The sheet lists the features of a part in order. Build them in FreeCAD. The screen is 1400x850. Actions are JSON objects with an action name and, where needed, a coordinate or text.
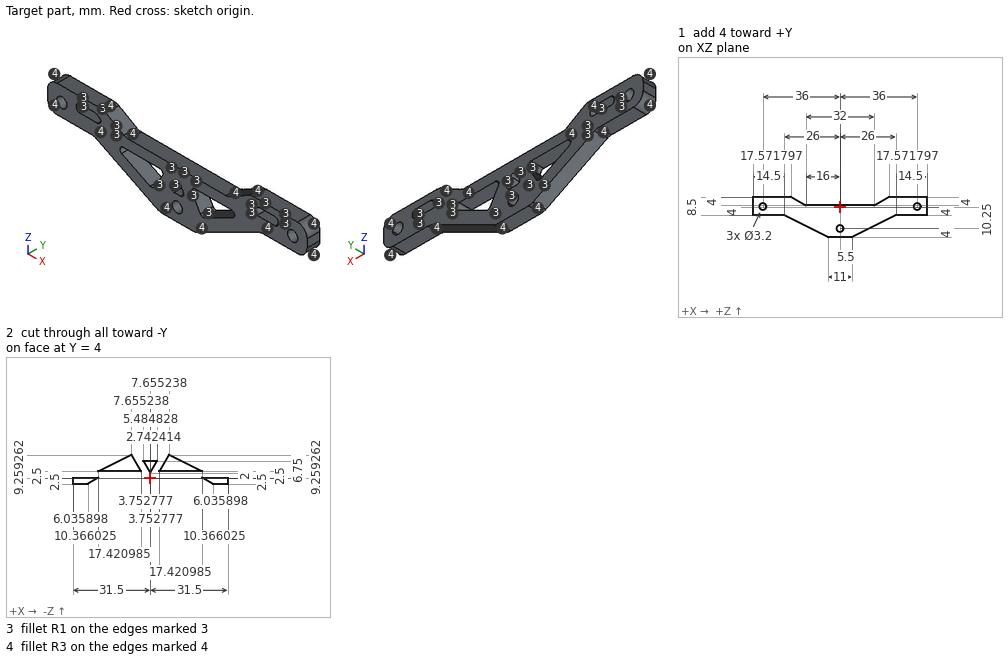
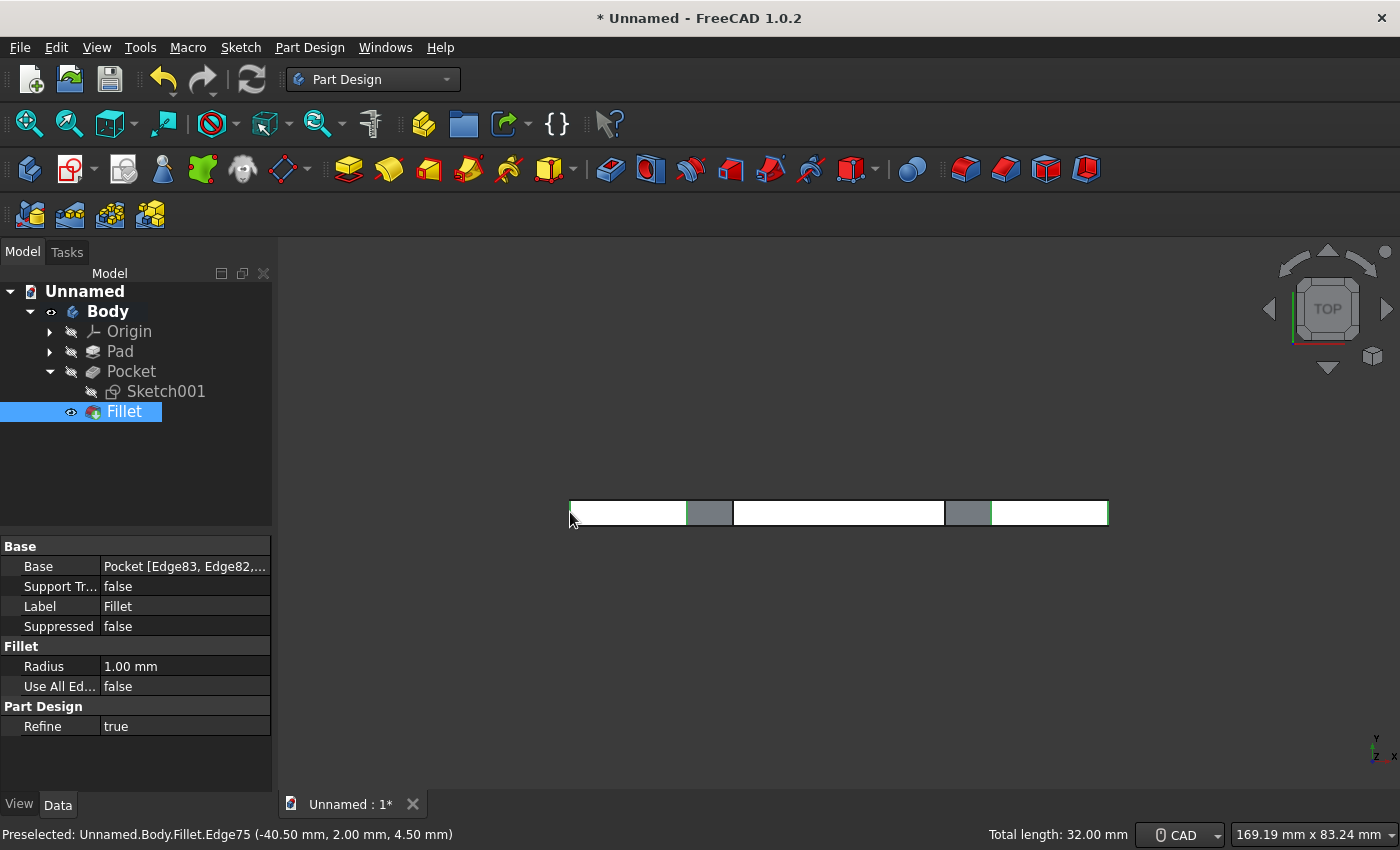
{"action": "key", "text": "1"}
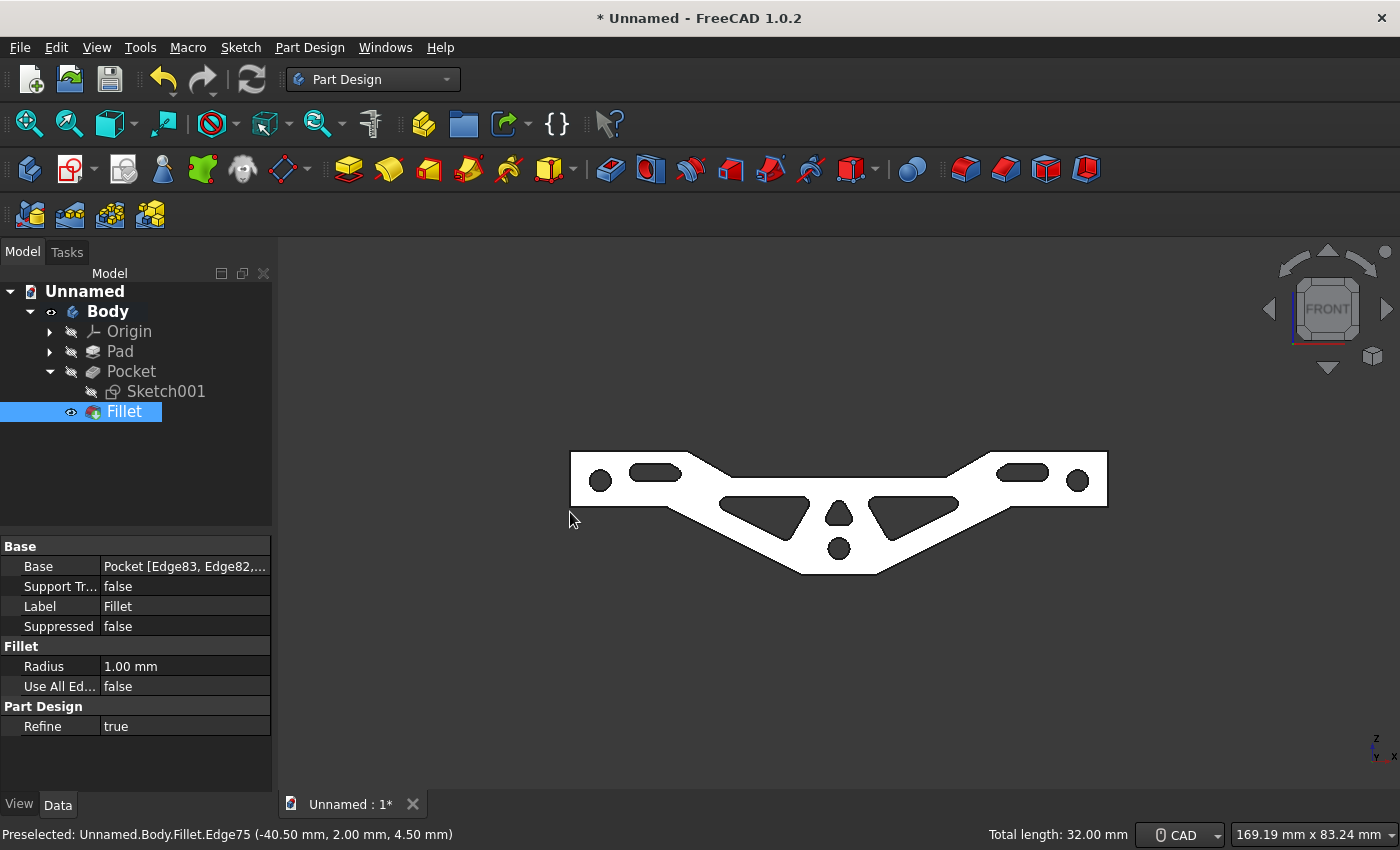
{"action": "key", "text": "3"}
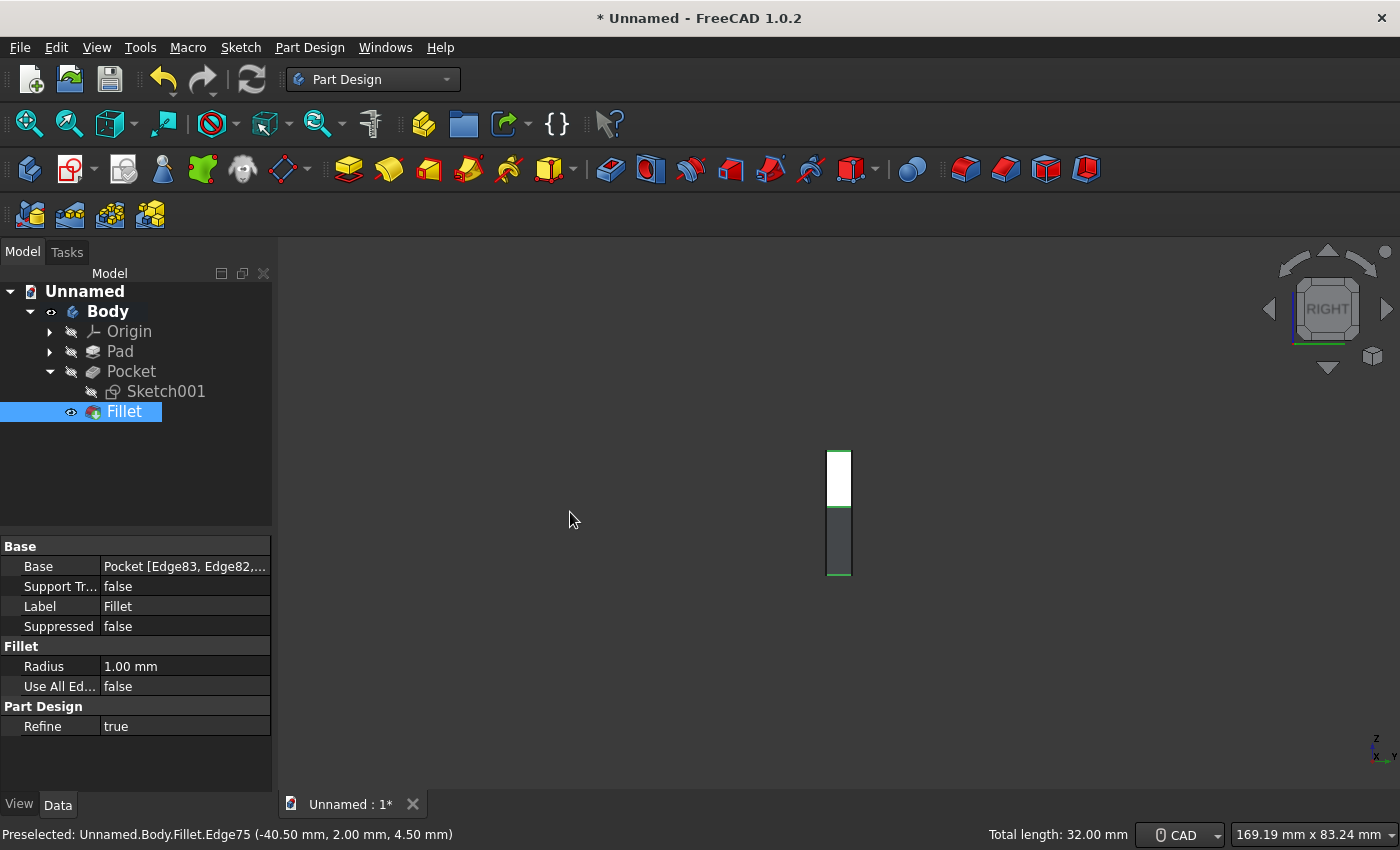
{"action": "left_click", "coordinate": [30, 124]}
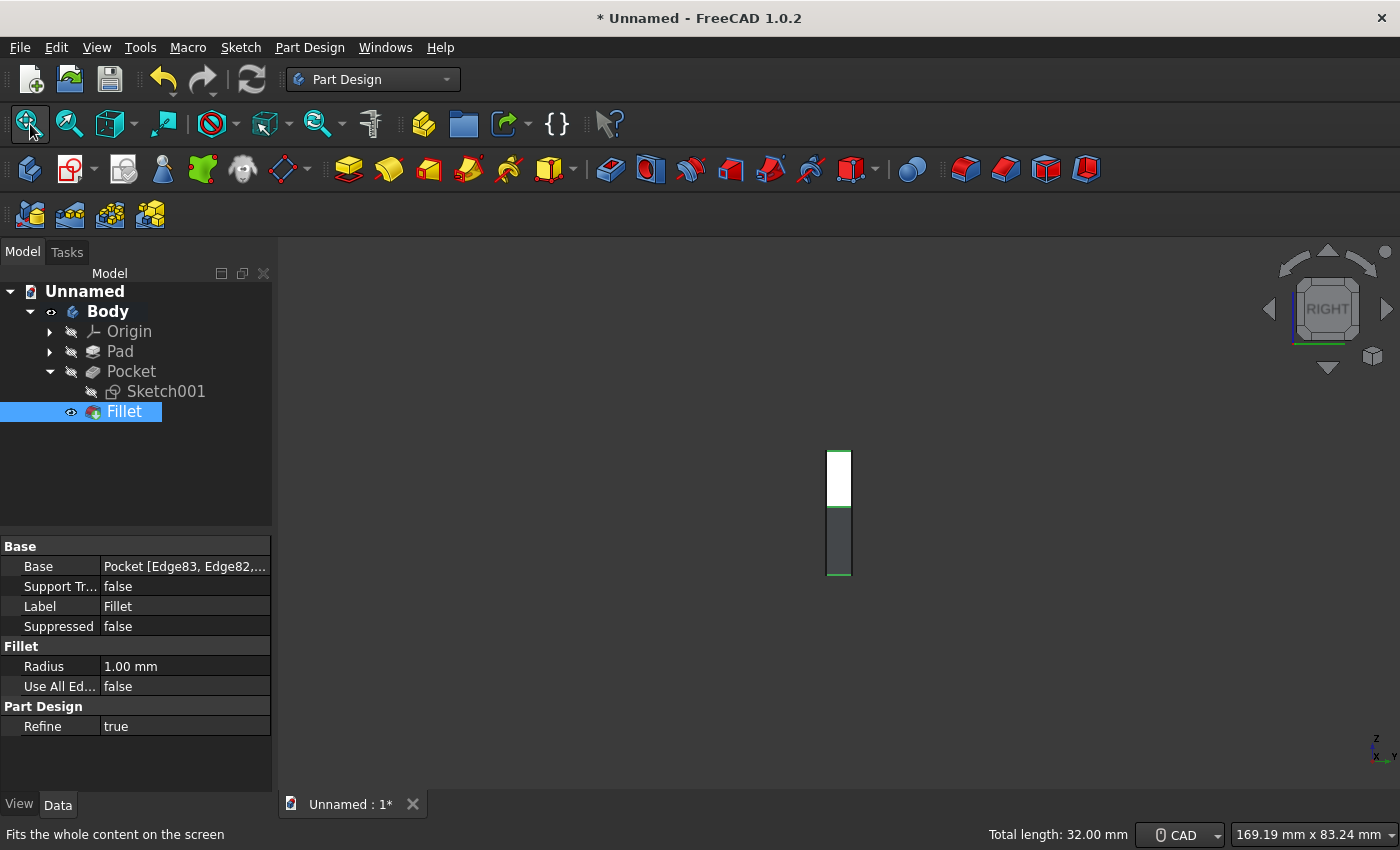
{"action": "key", "text": "5"}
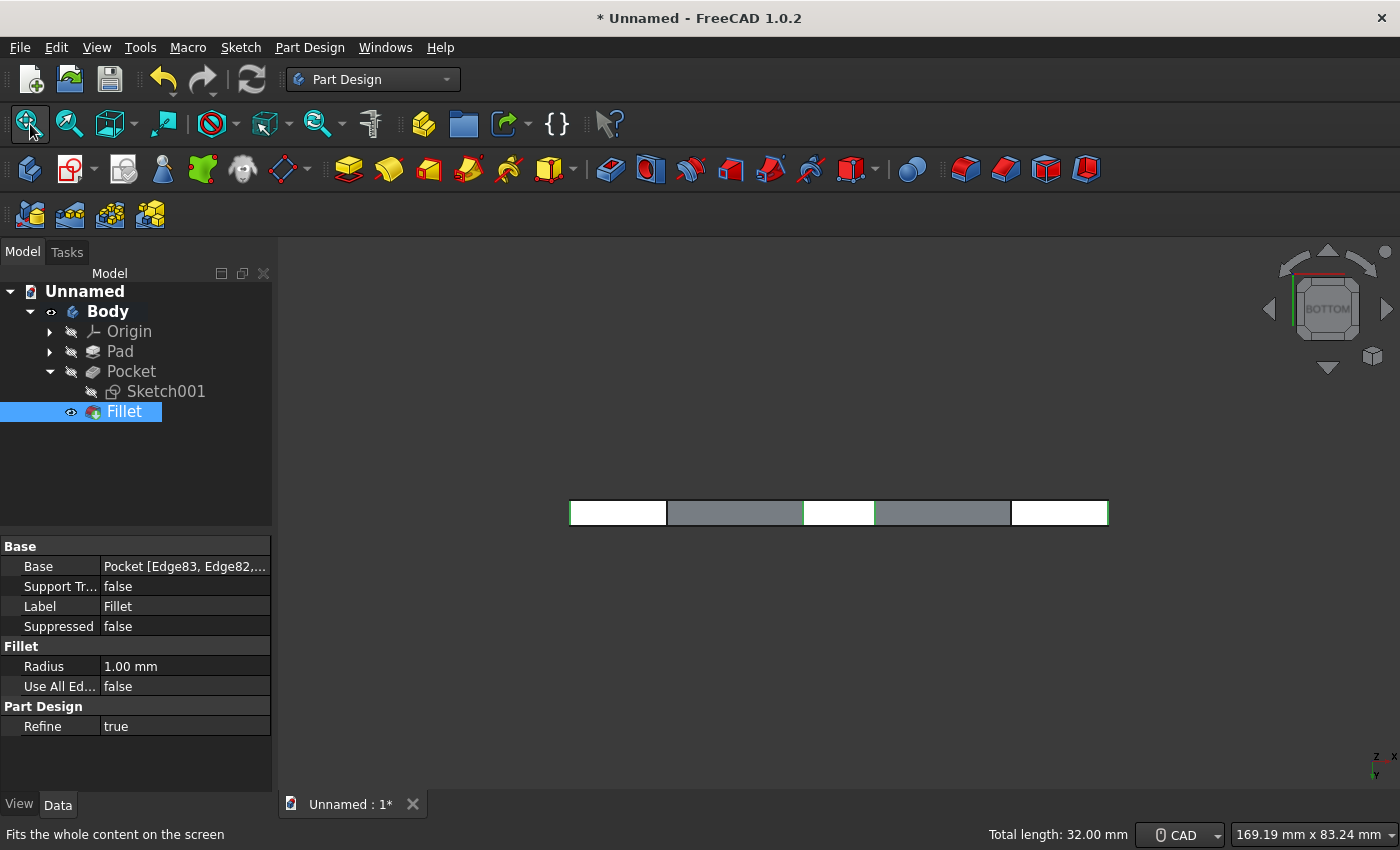
{"action": "key", "text": "4"}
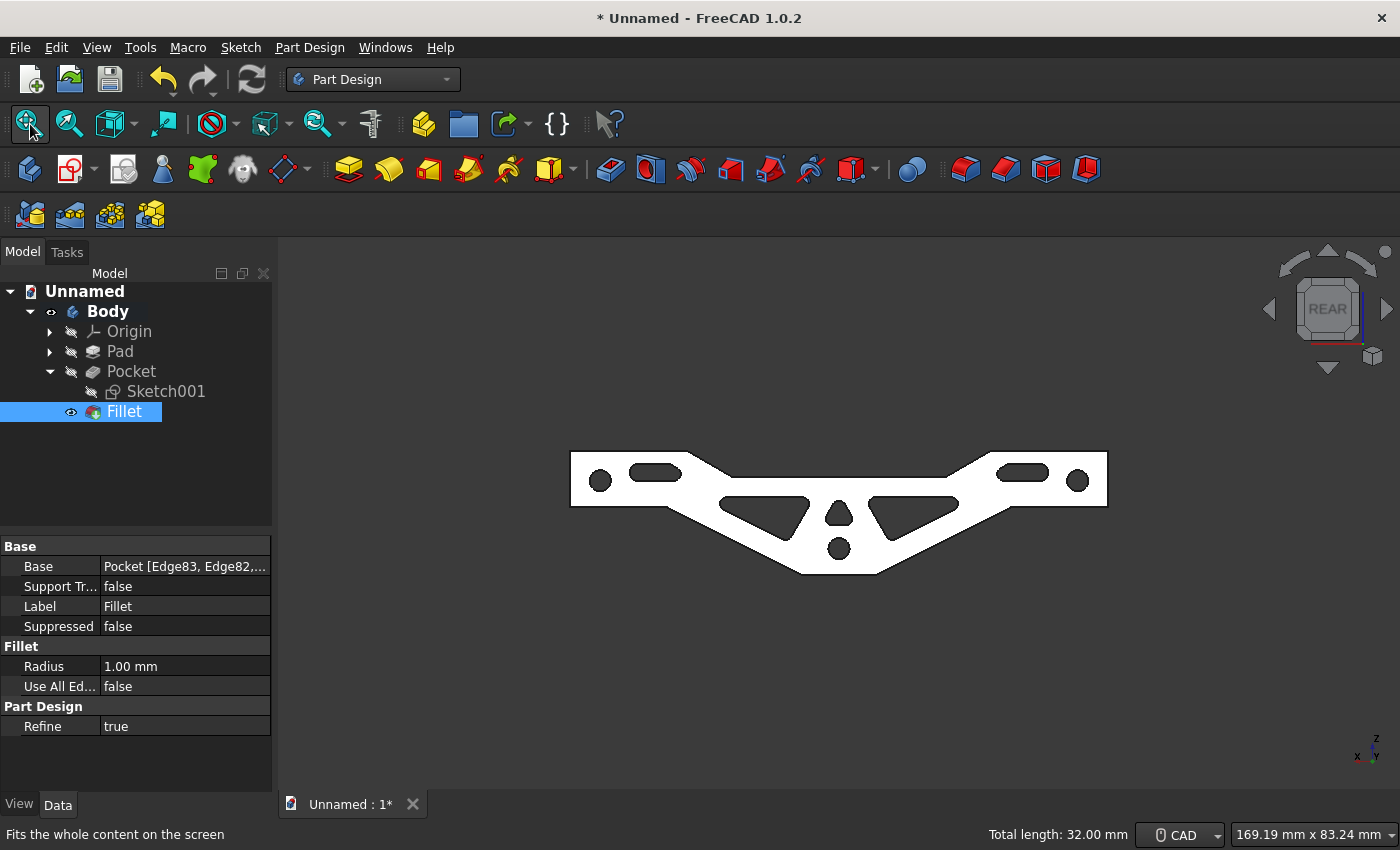
{"action": "key", "text": "6"}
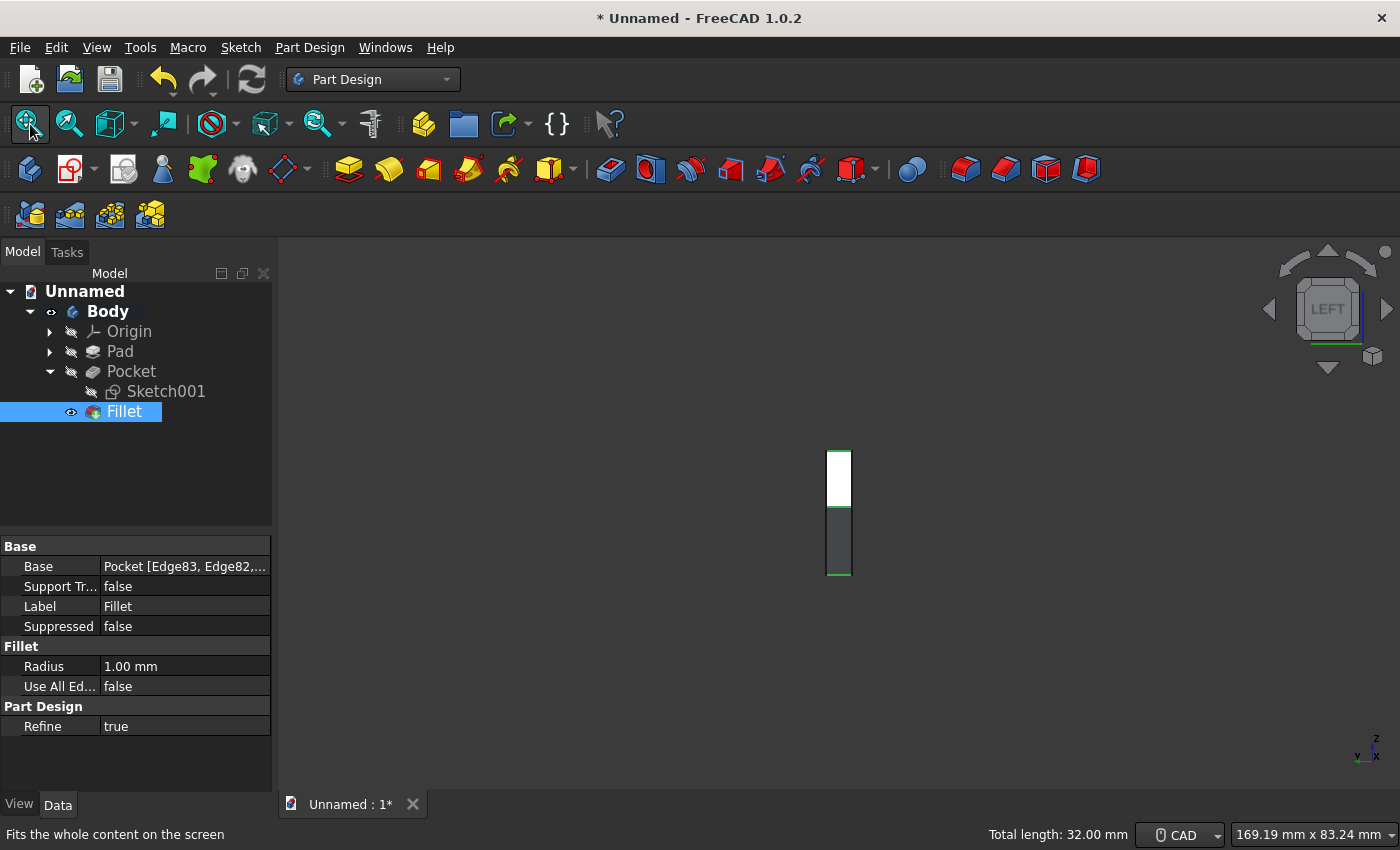
{"action": "left_click", "coordinate": [30, 124]}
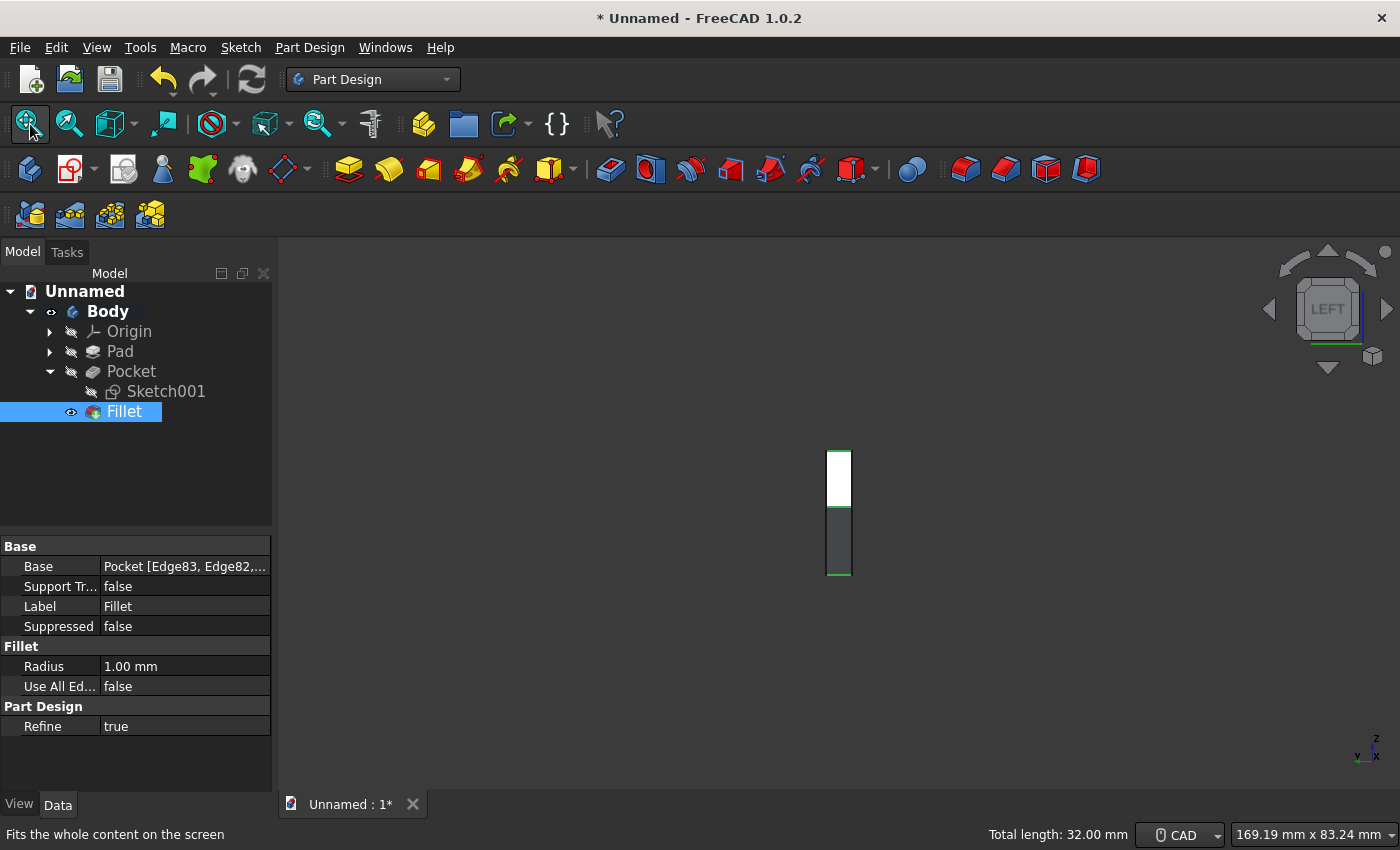
{"action": "key", "text": "v 3"}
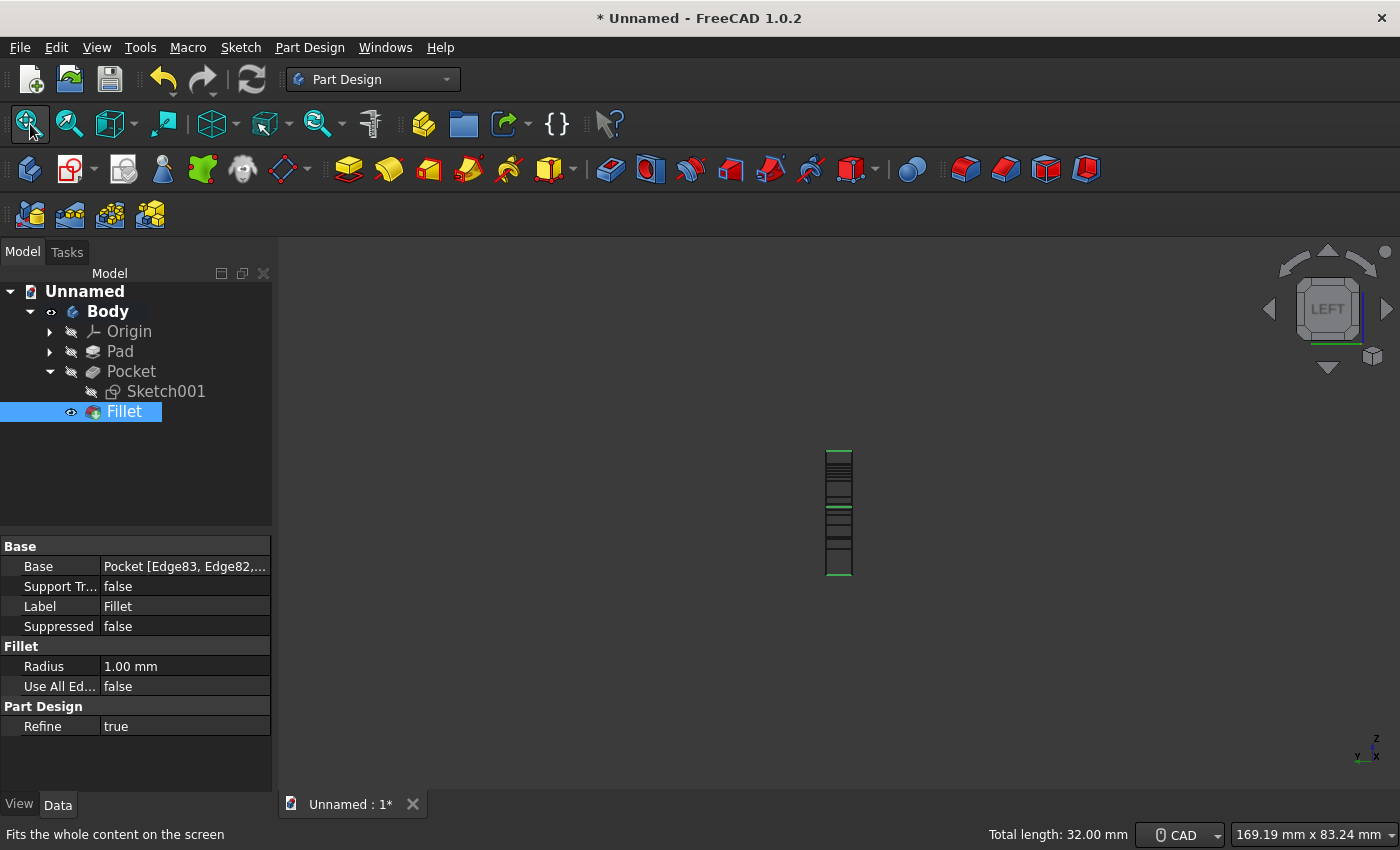
{"action": "key", "text": "0"}